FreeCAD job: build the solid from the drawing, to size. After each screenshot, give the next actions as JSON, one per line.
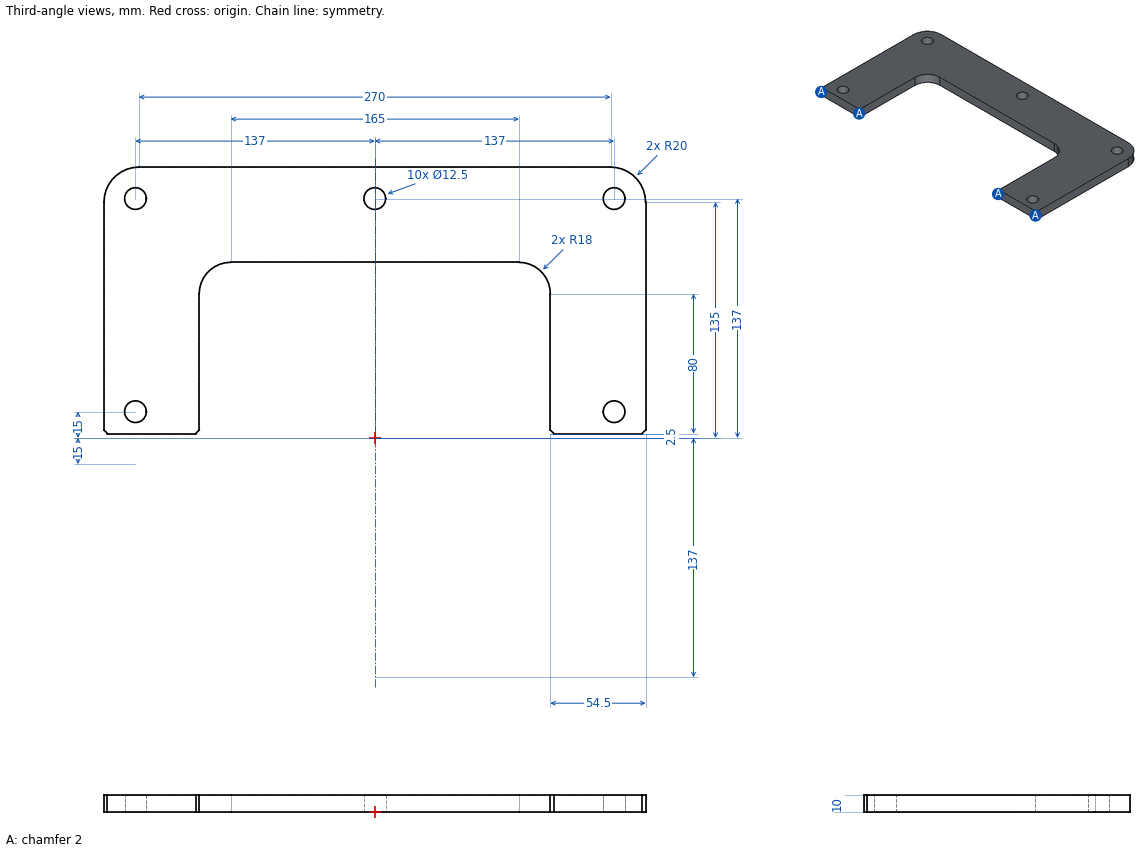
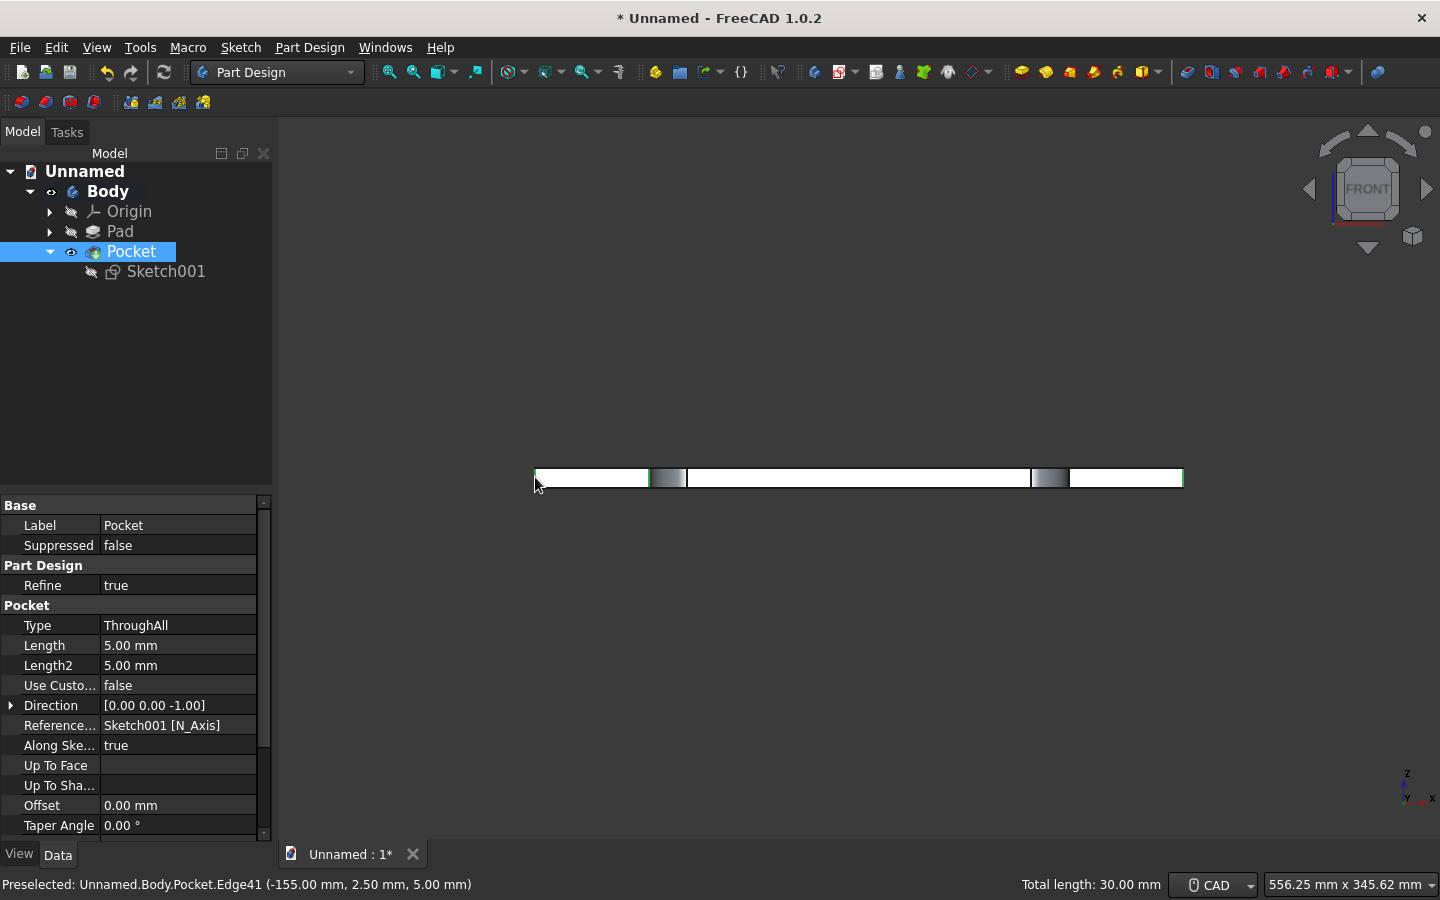
{"action": "left_click", "coordinate": [1069, 477], "text": "ctrl"}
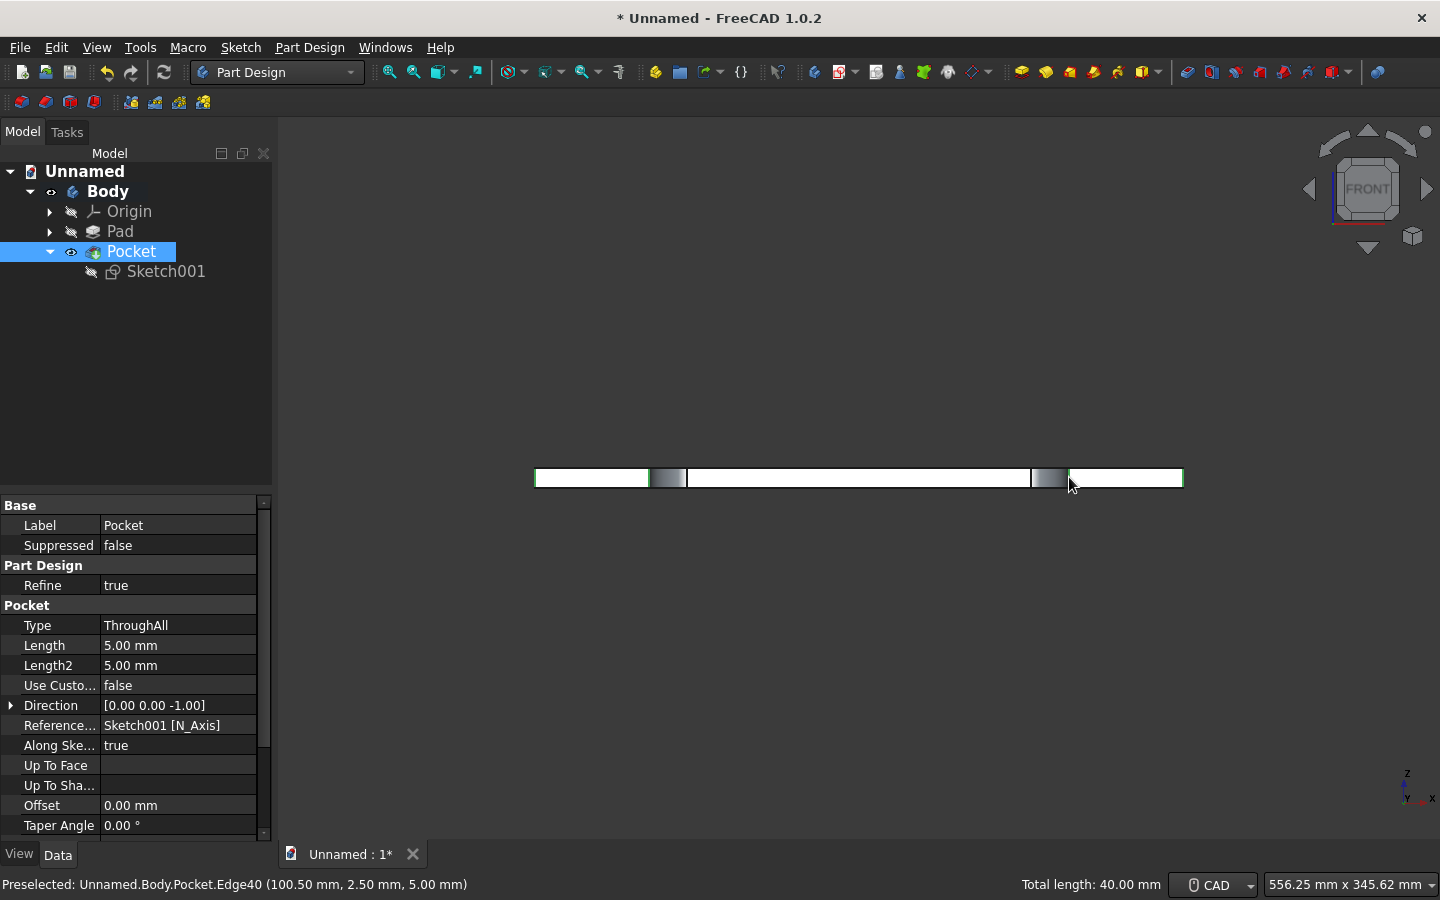
{"action": "left_click", "coordinate": [46, 102]}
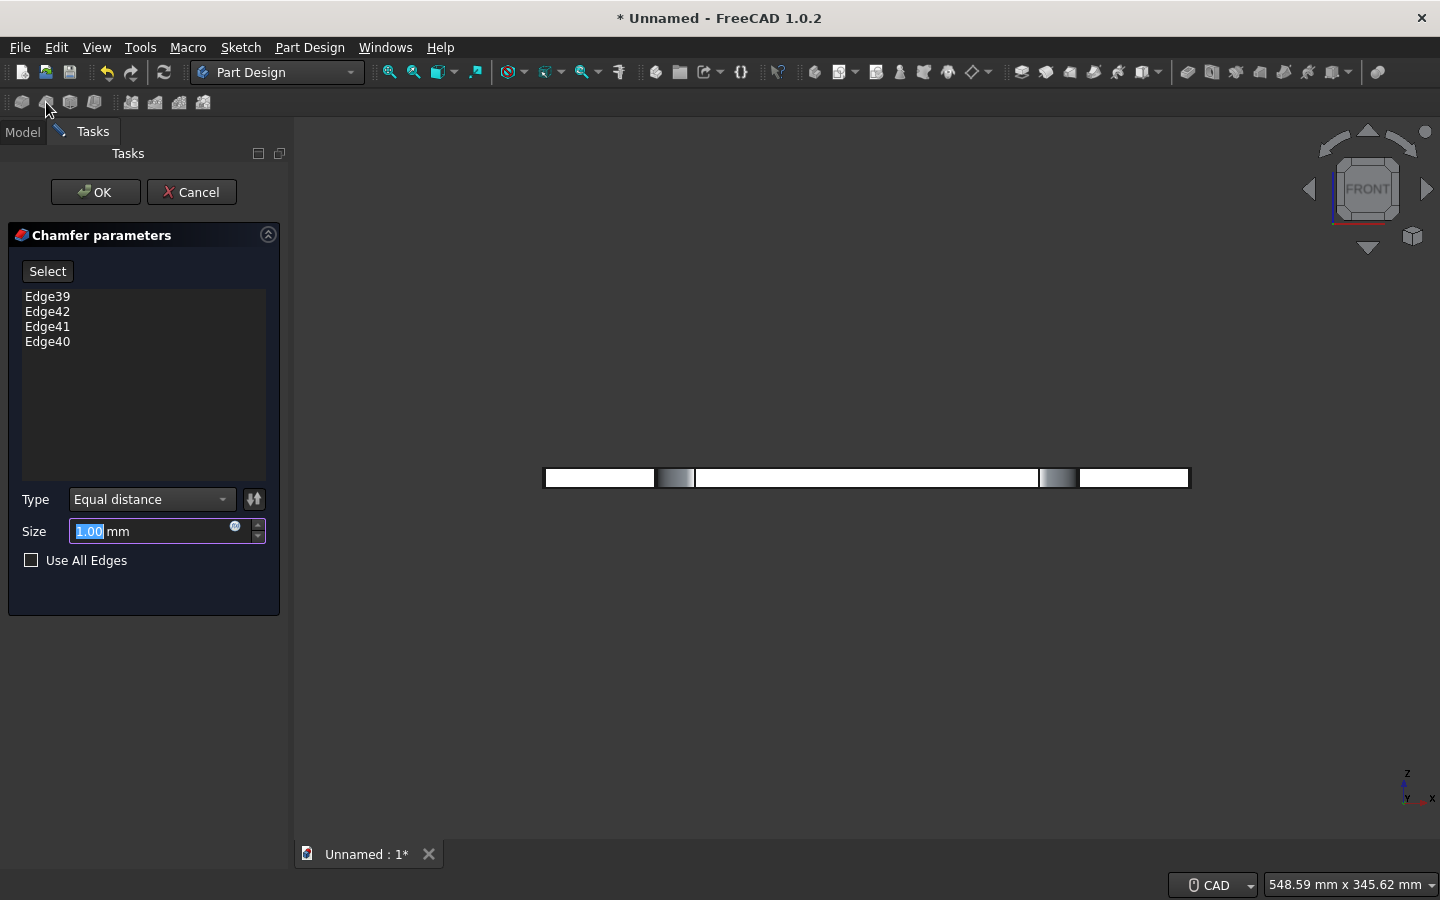
{"action": "type", "text": "2"}
{"action": "key", "text": "Tab"}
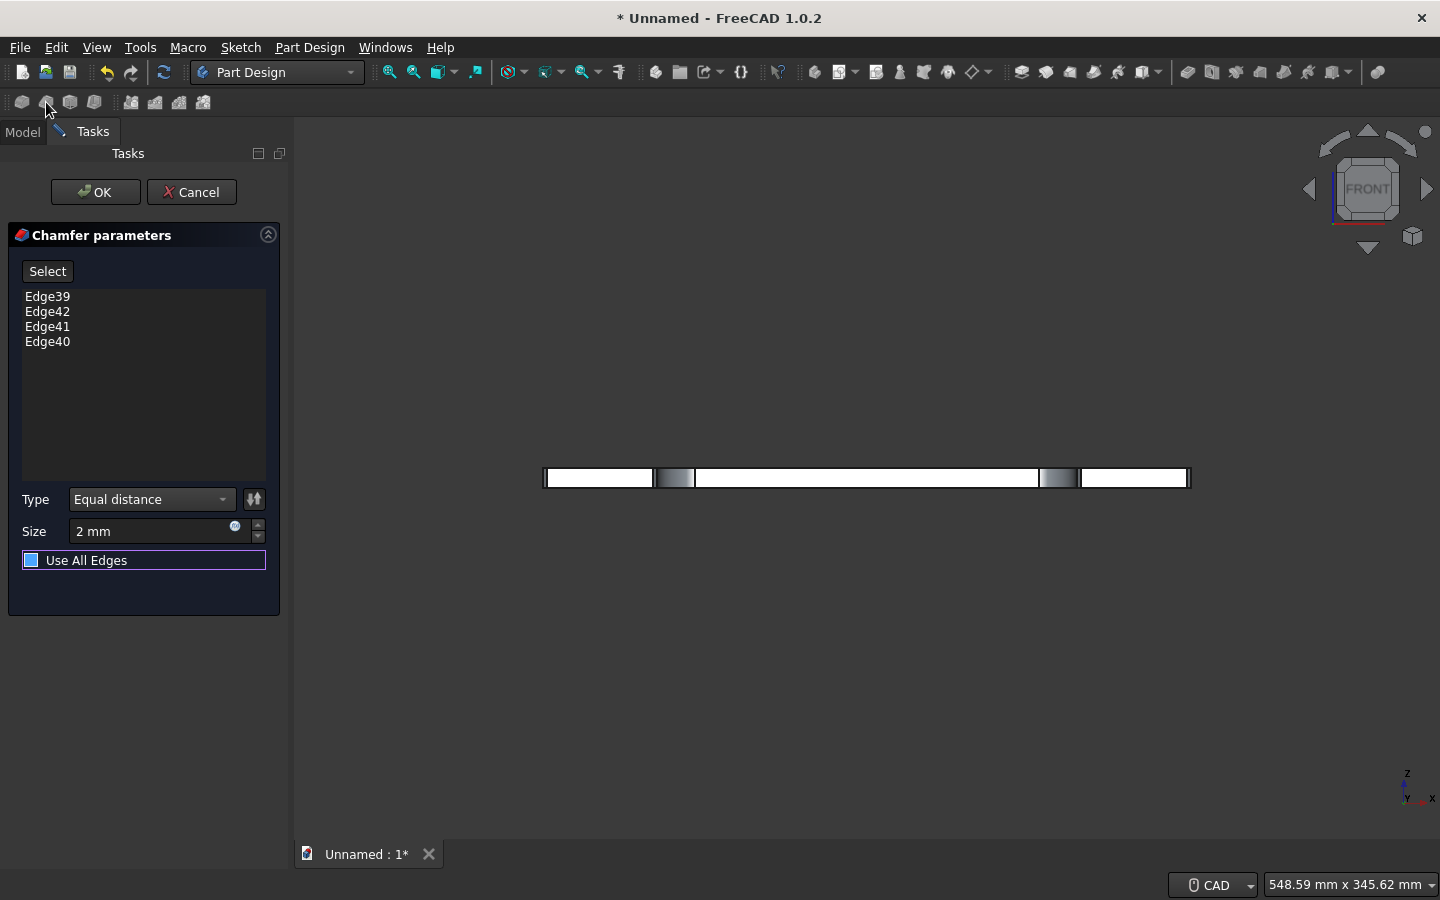
{"action": "left_click", "coordinate": [96, 192]}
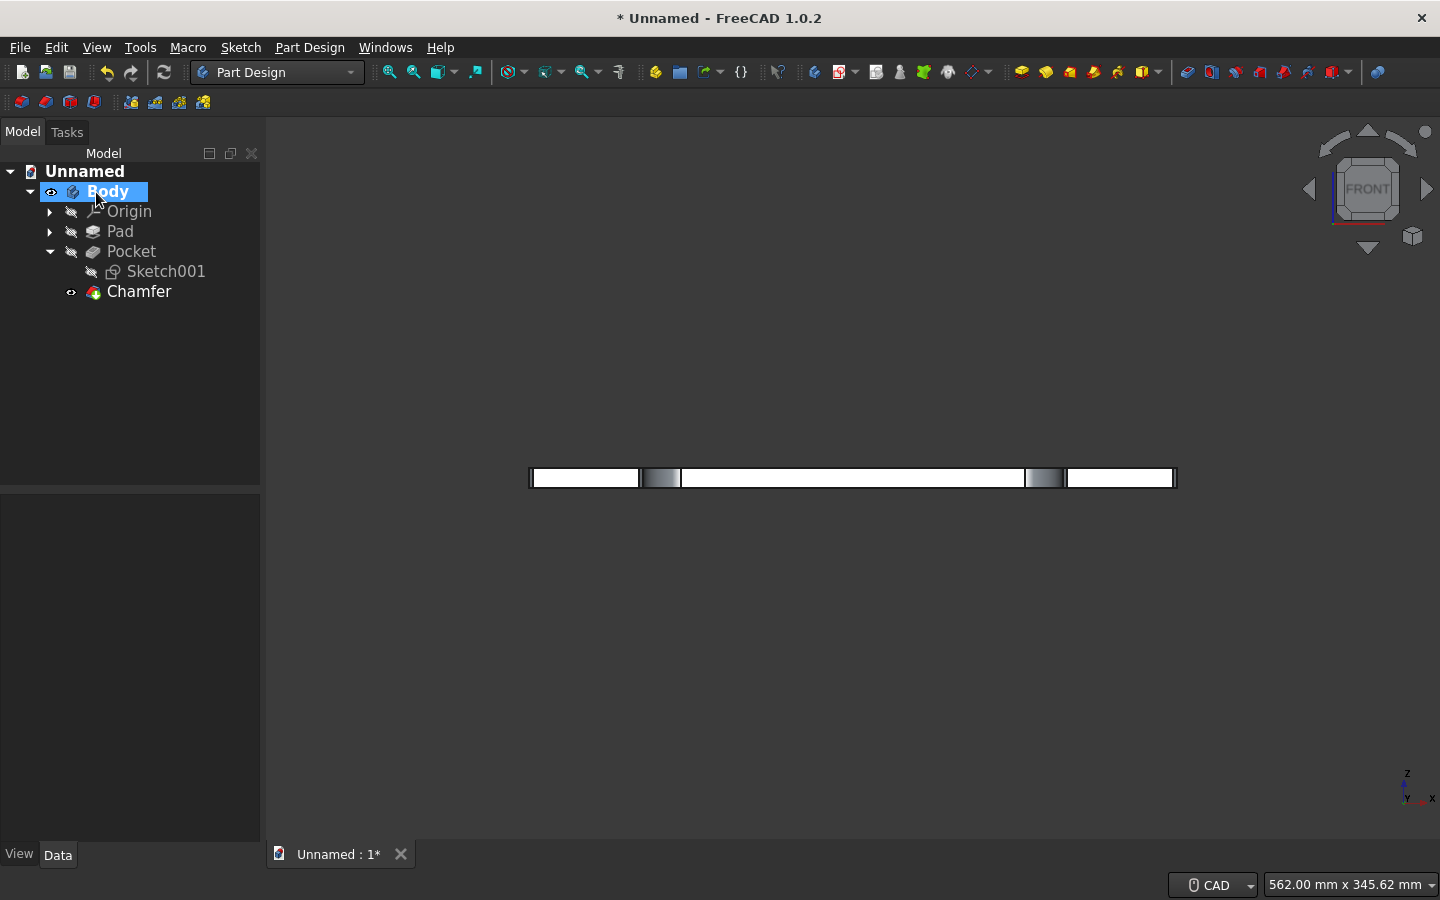
{"action": "key", "text": "0"}